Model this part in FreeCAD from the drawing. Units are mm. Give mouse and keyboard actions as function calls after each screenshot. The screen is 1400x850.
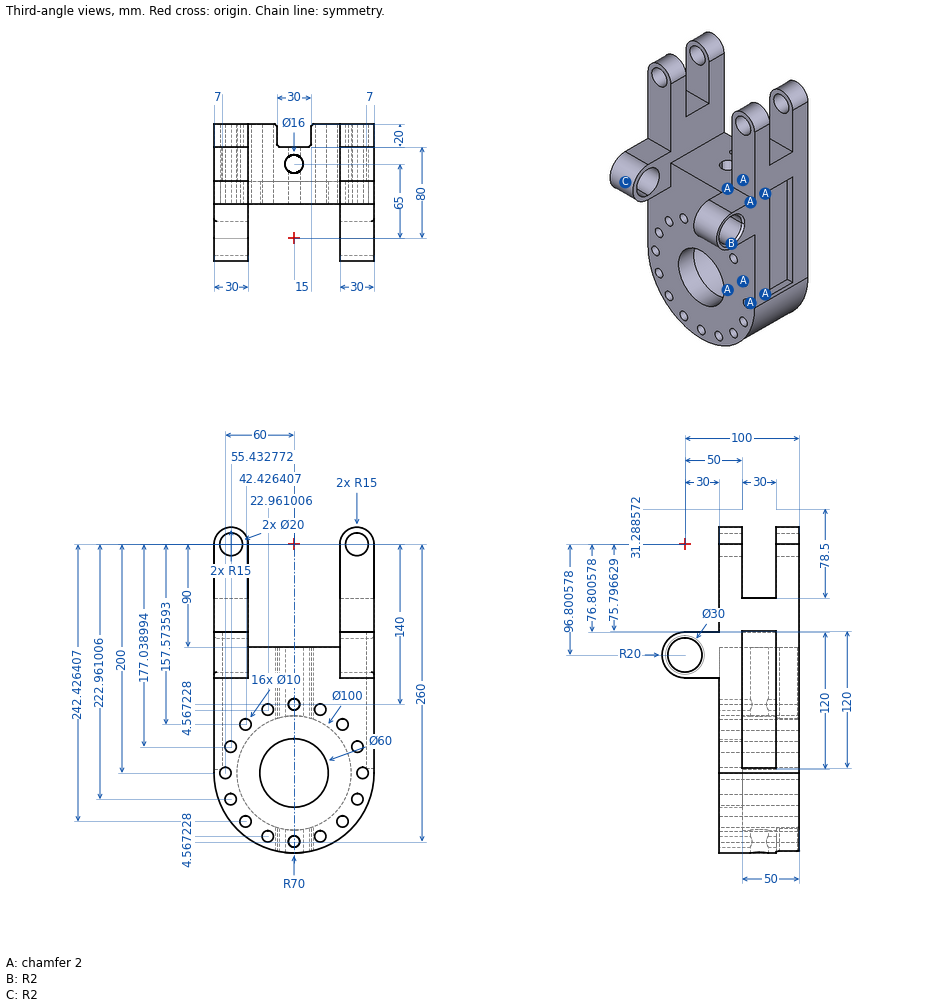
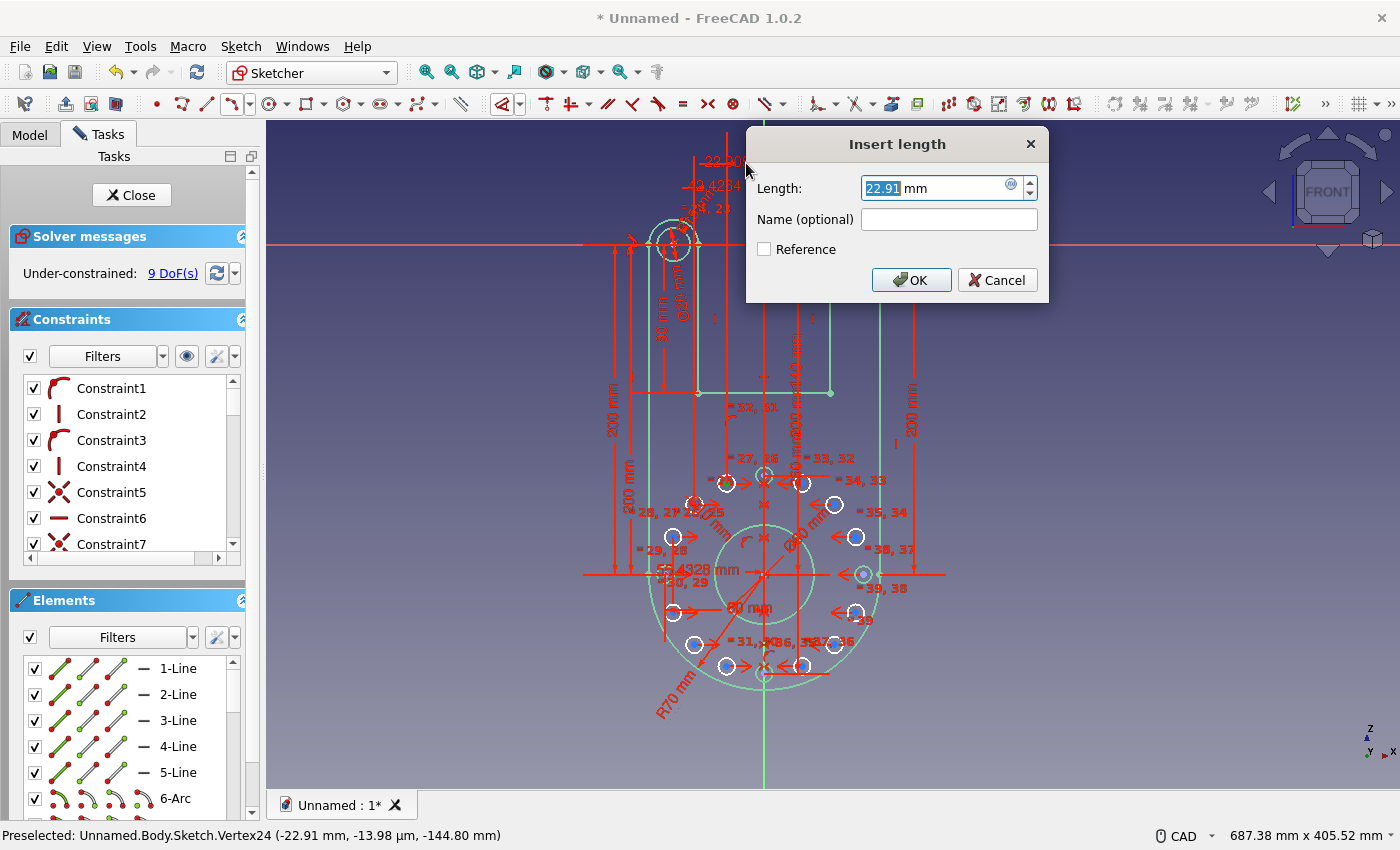
text(22.961006)
key(Return)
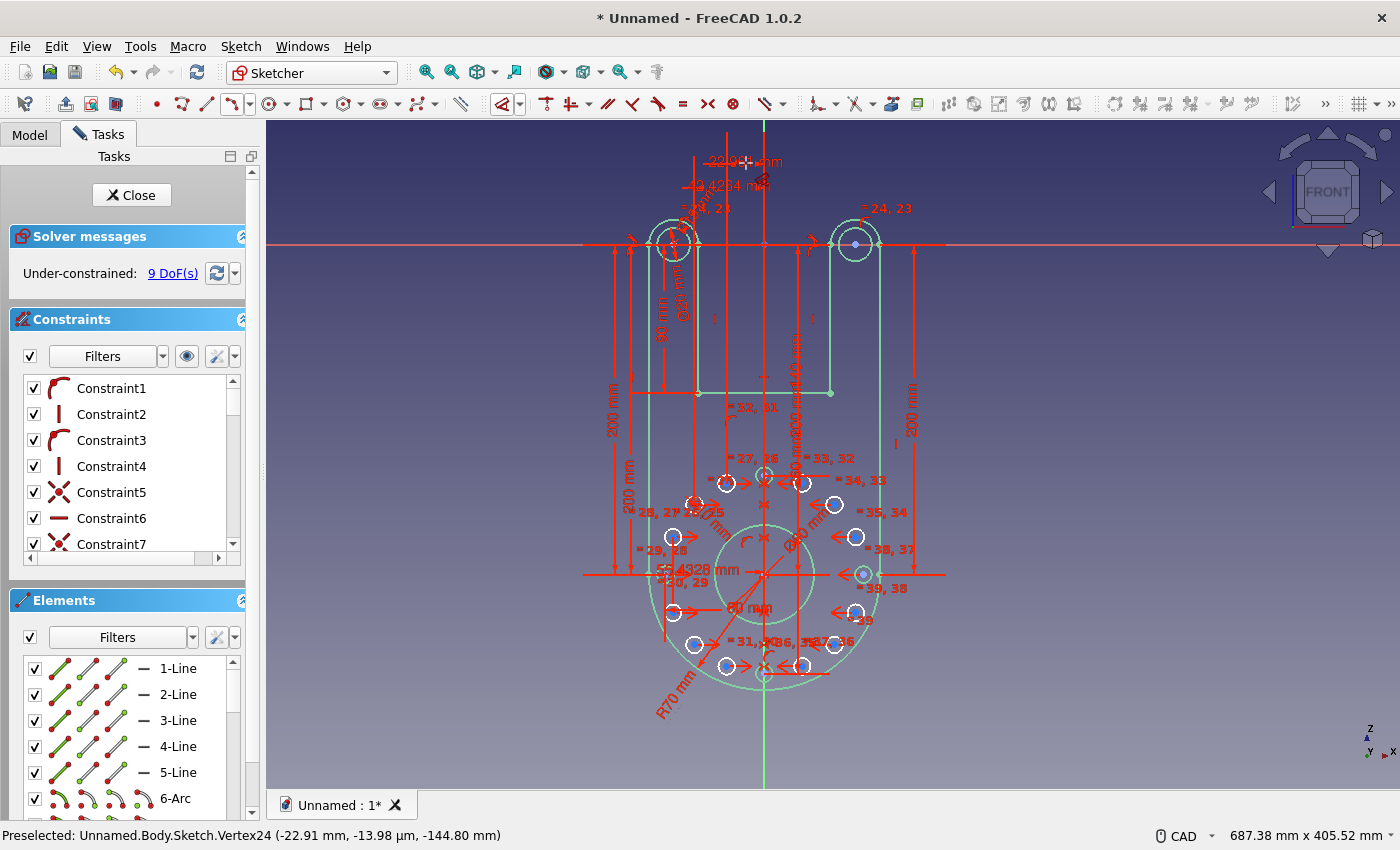
click(673, 613)
click(740, 647)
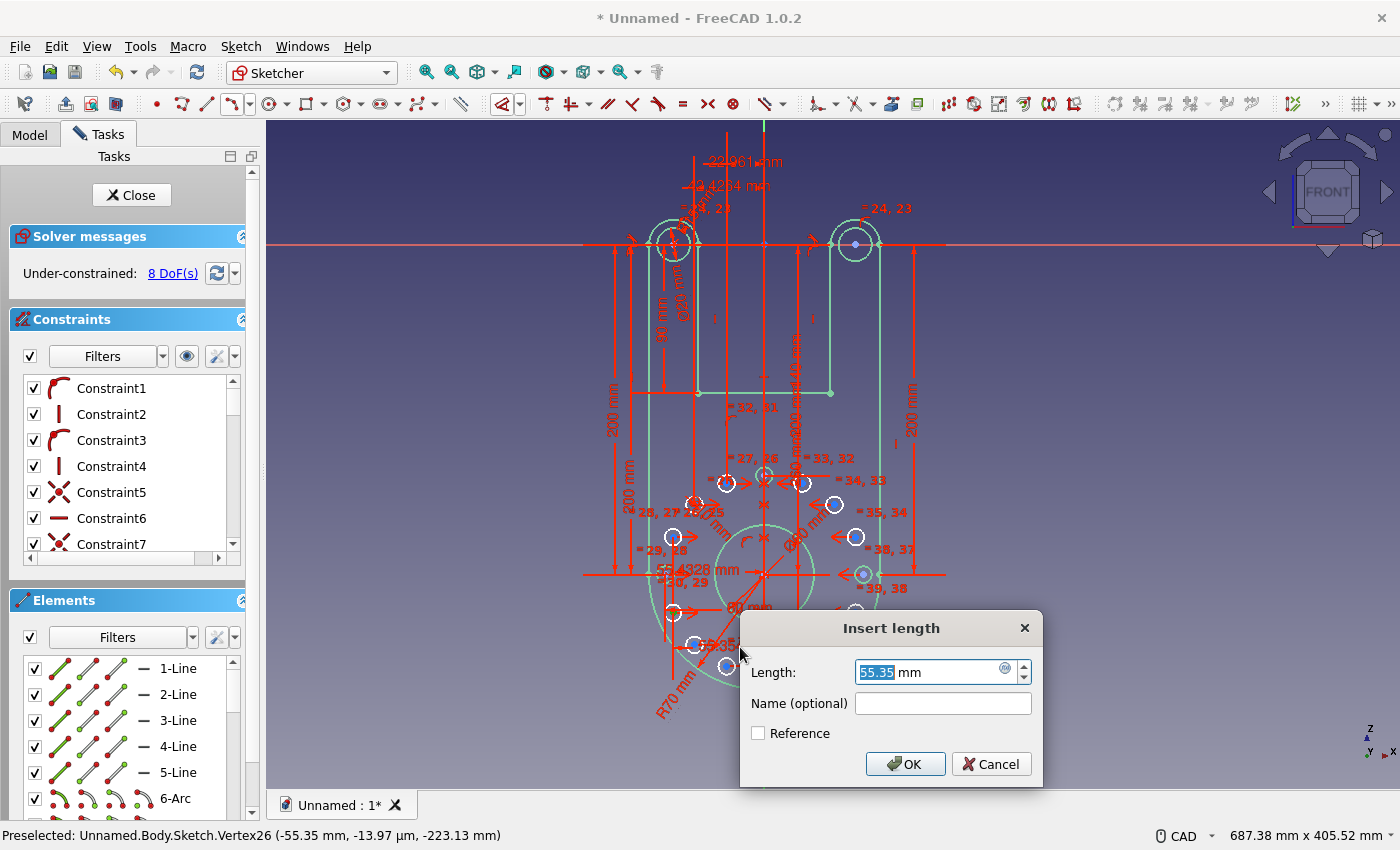
text(55.432772)
key(Return)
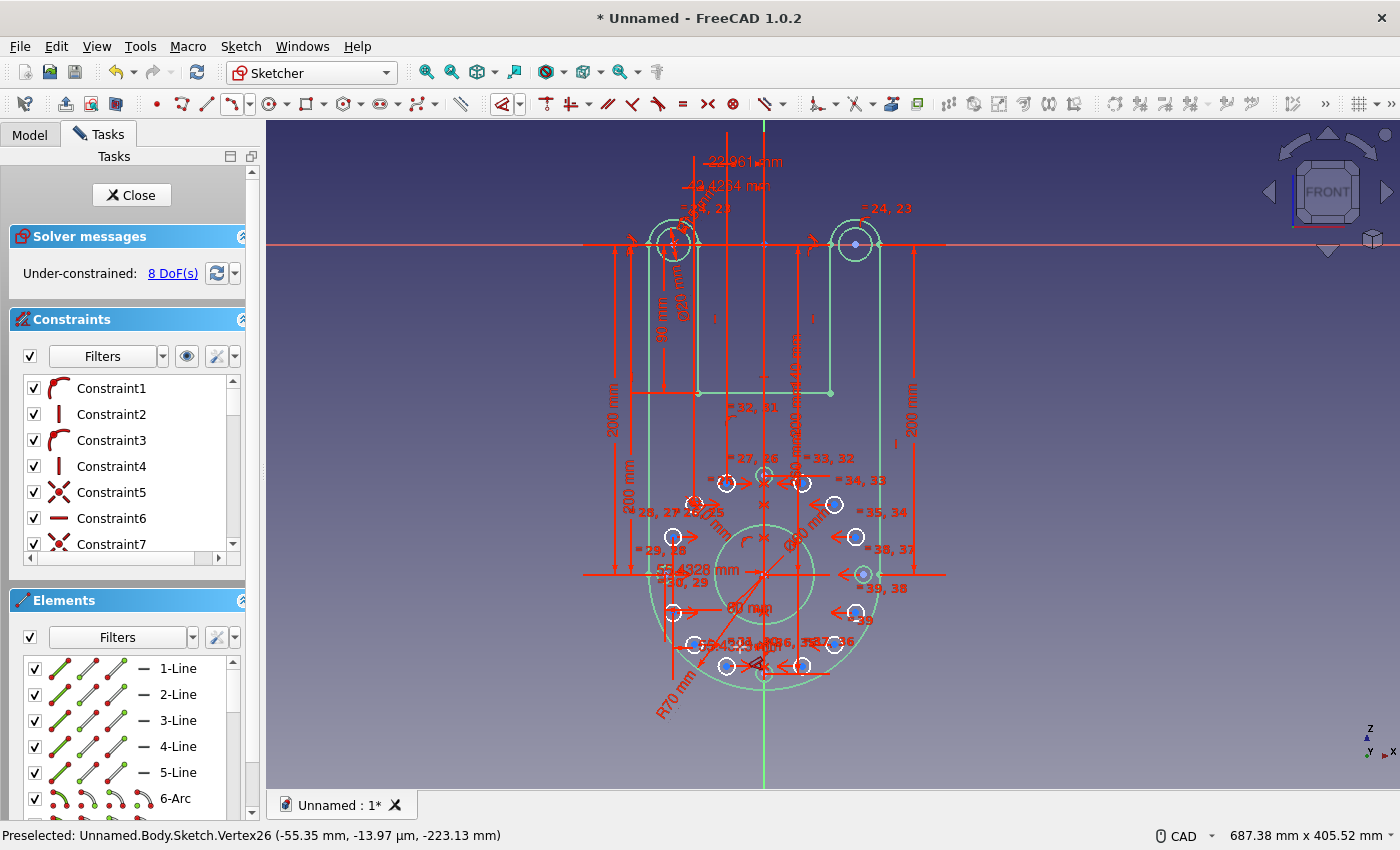
click(694, 645)
click(729, 727)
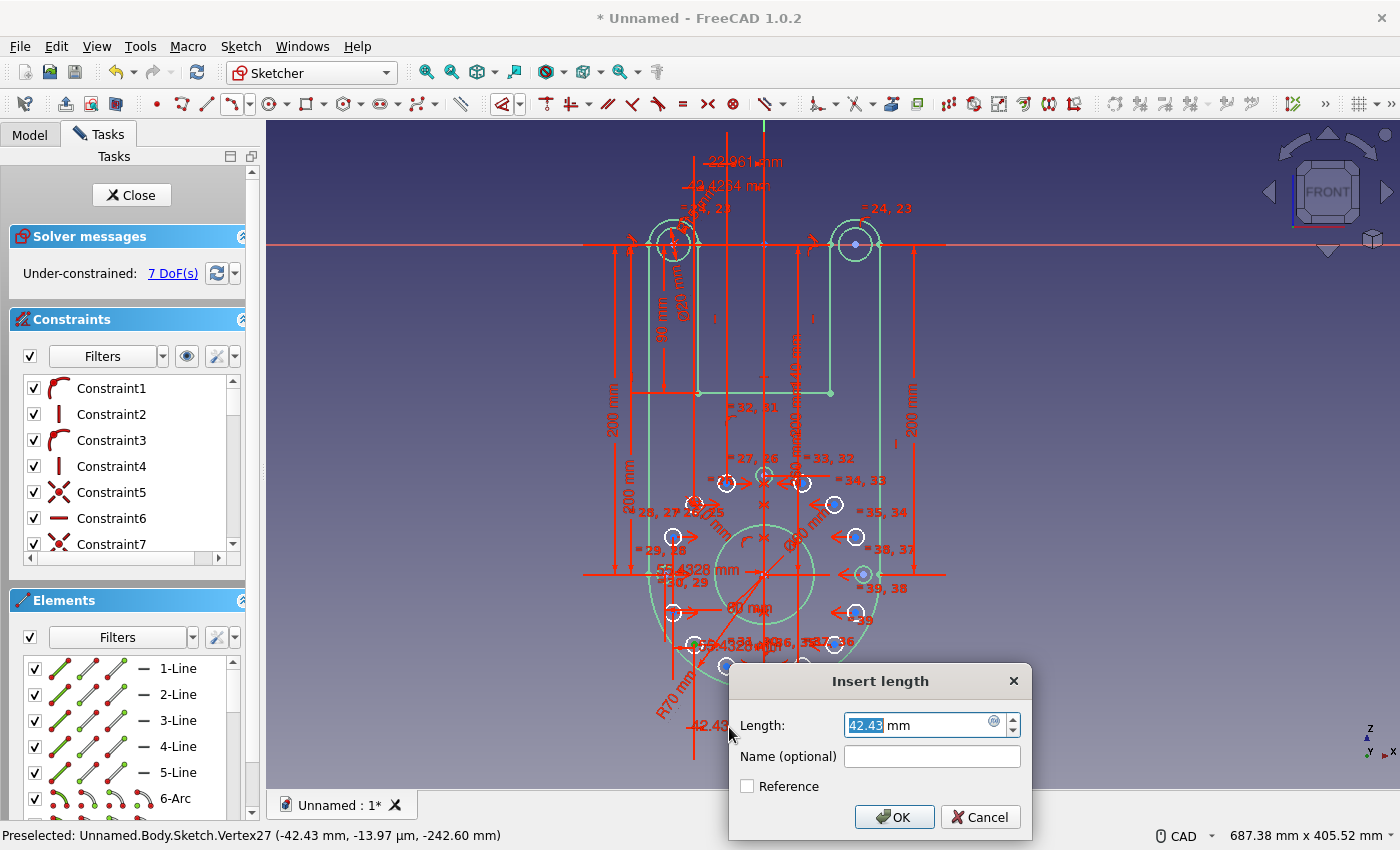
text(42.426407)
key(Return)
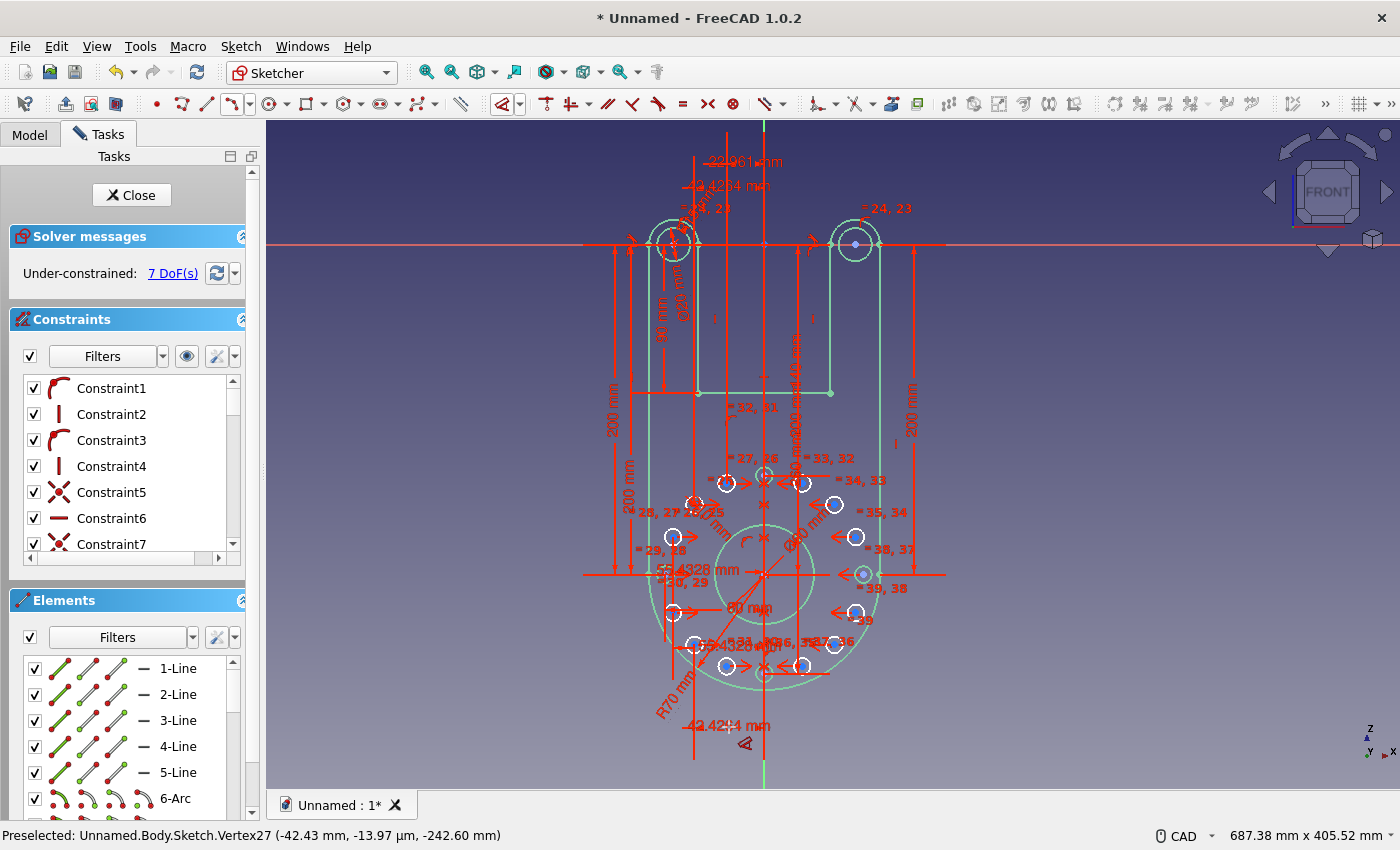
click(727, 666)
click(746, 748)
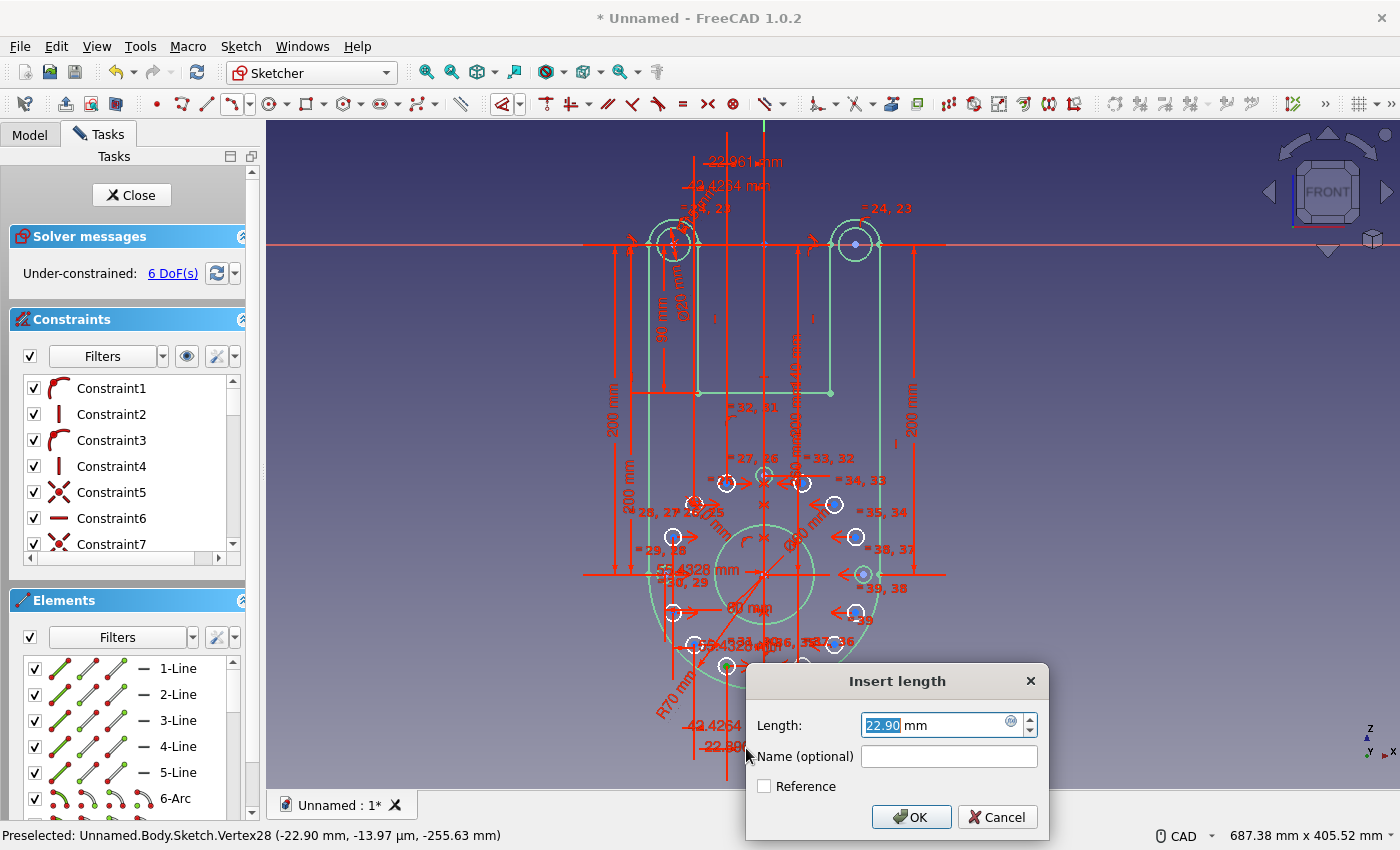
text(22.961006)
key(Return)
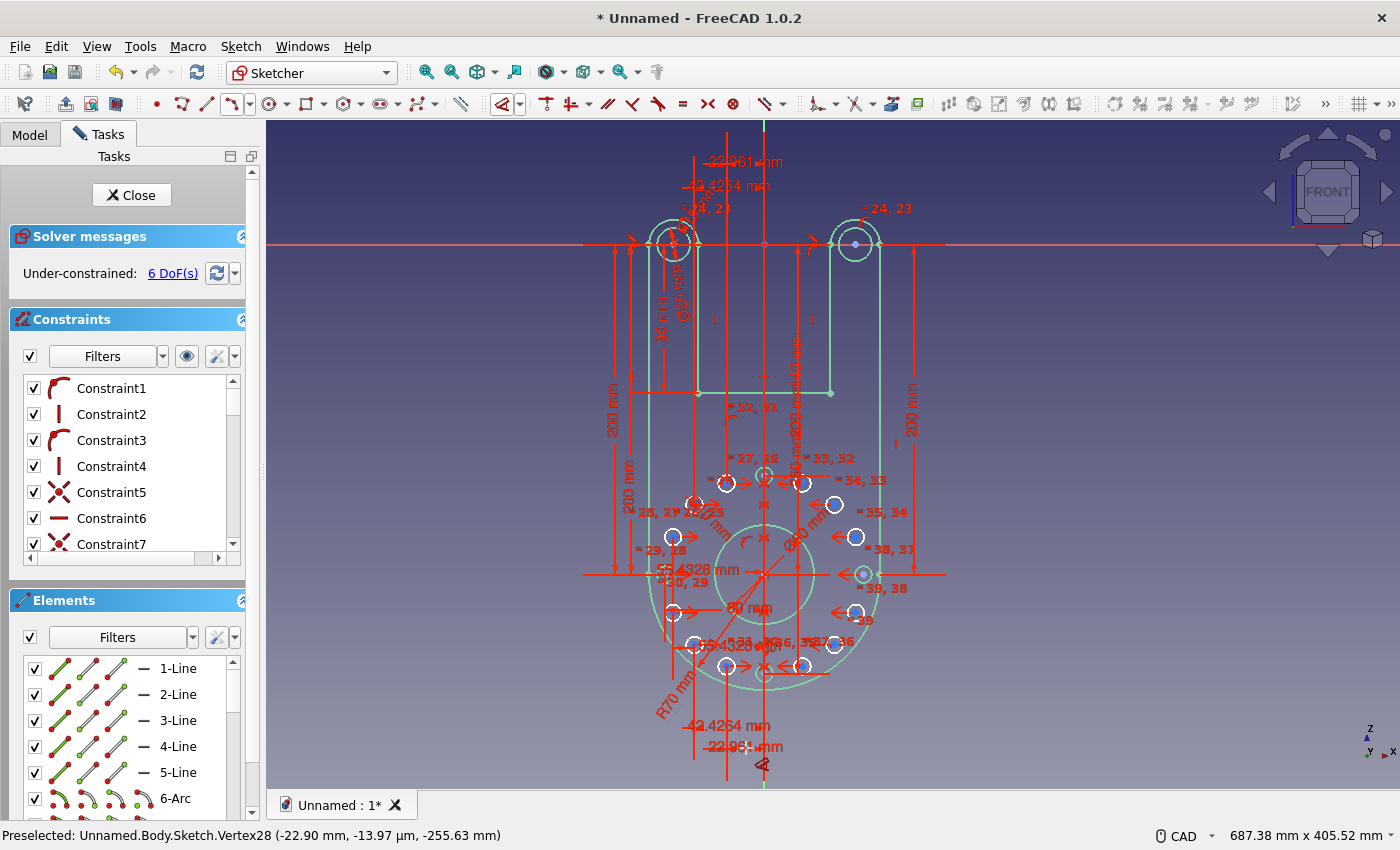
scroll(727, 484, up, 9)